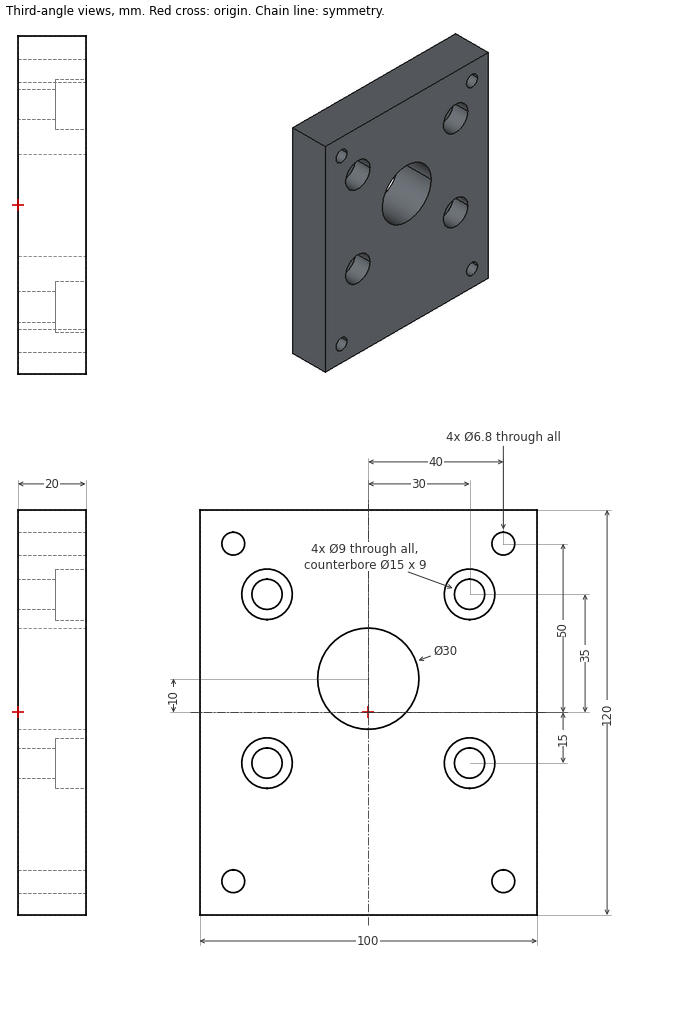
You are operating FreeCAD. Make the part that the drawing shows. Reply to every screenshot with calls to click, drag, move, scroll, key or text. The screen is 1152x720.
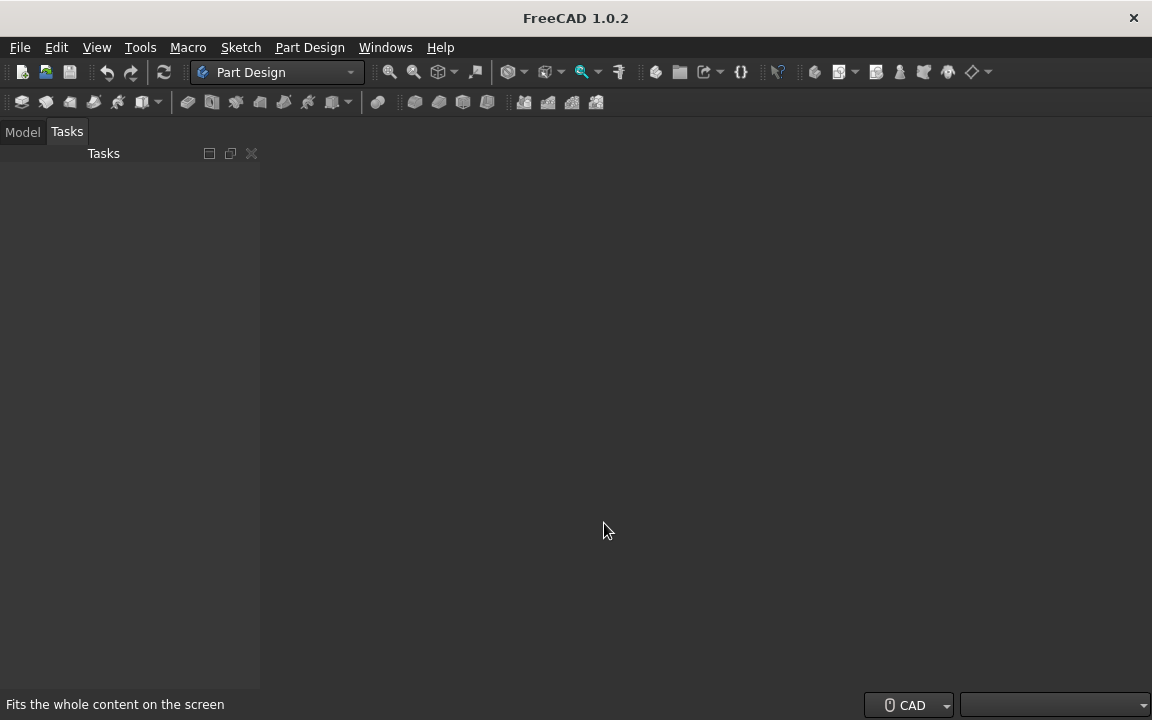
click(22, 72)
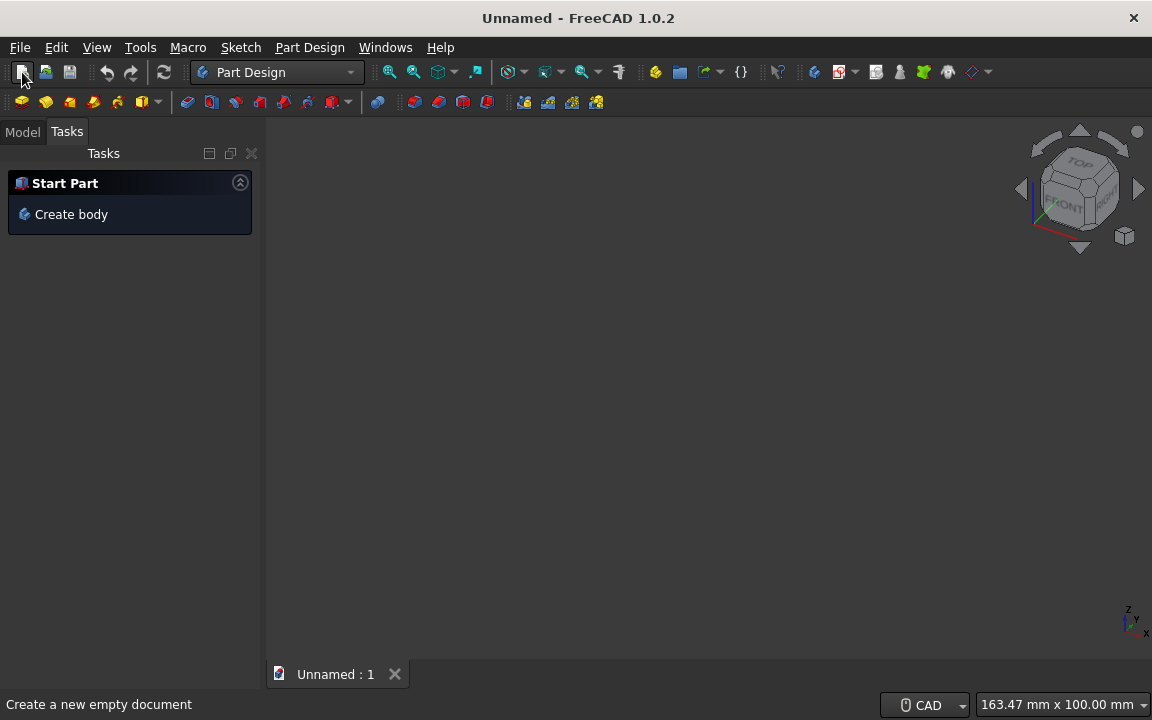
click(840, 72)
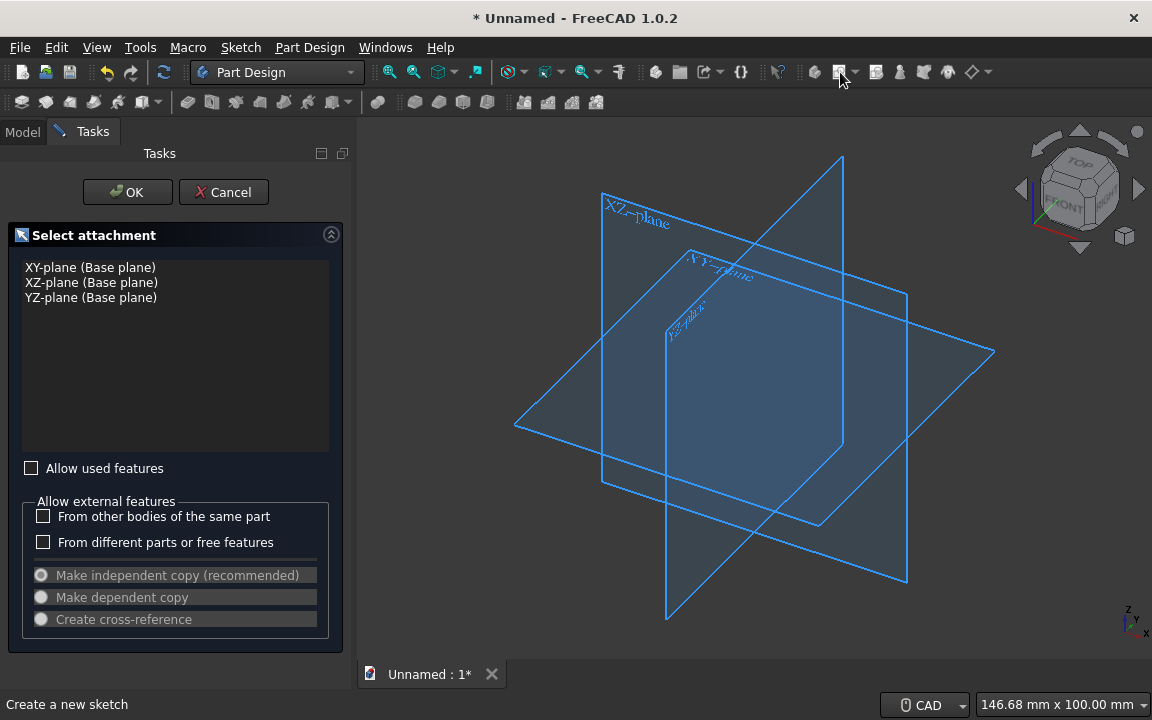
click(82, 298)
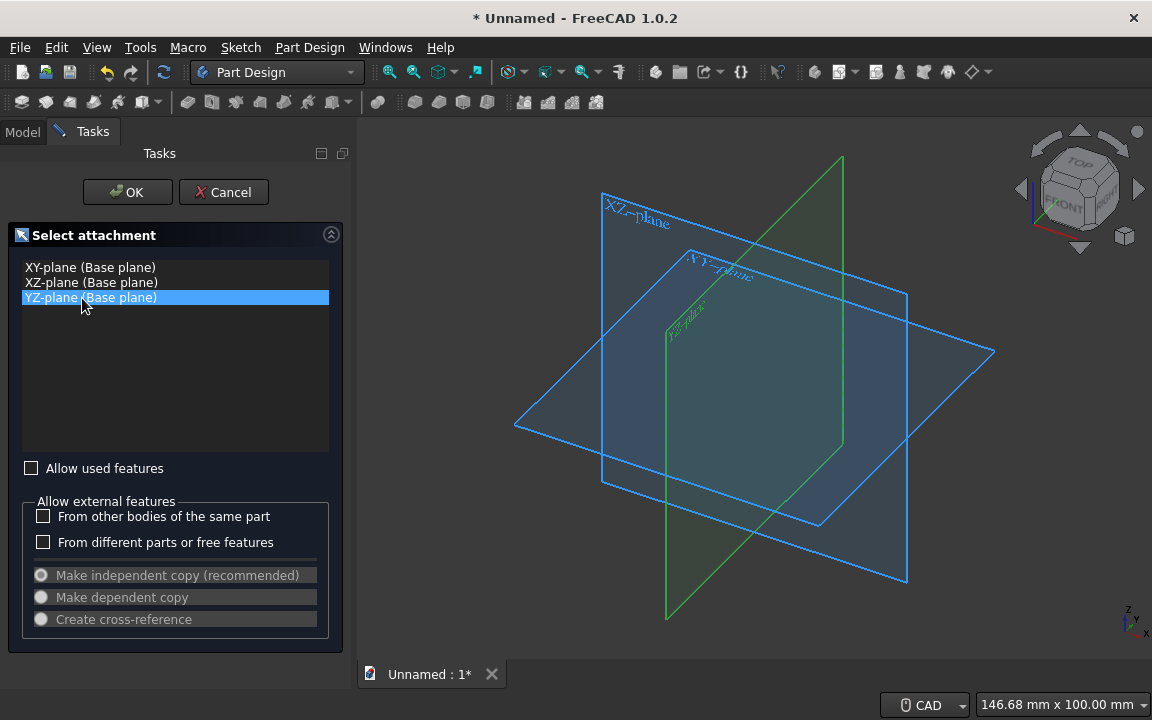
click(128, 192)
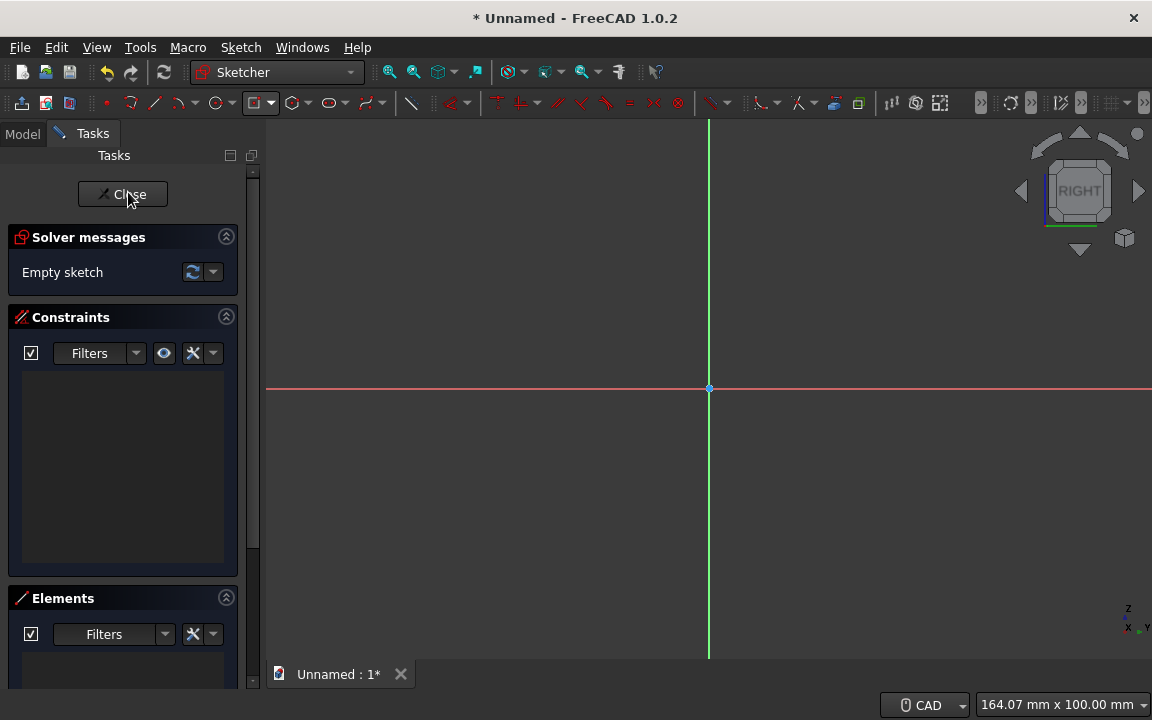
scroll(557, 389, down, 3)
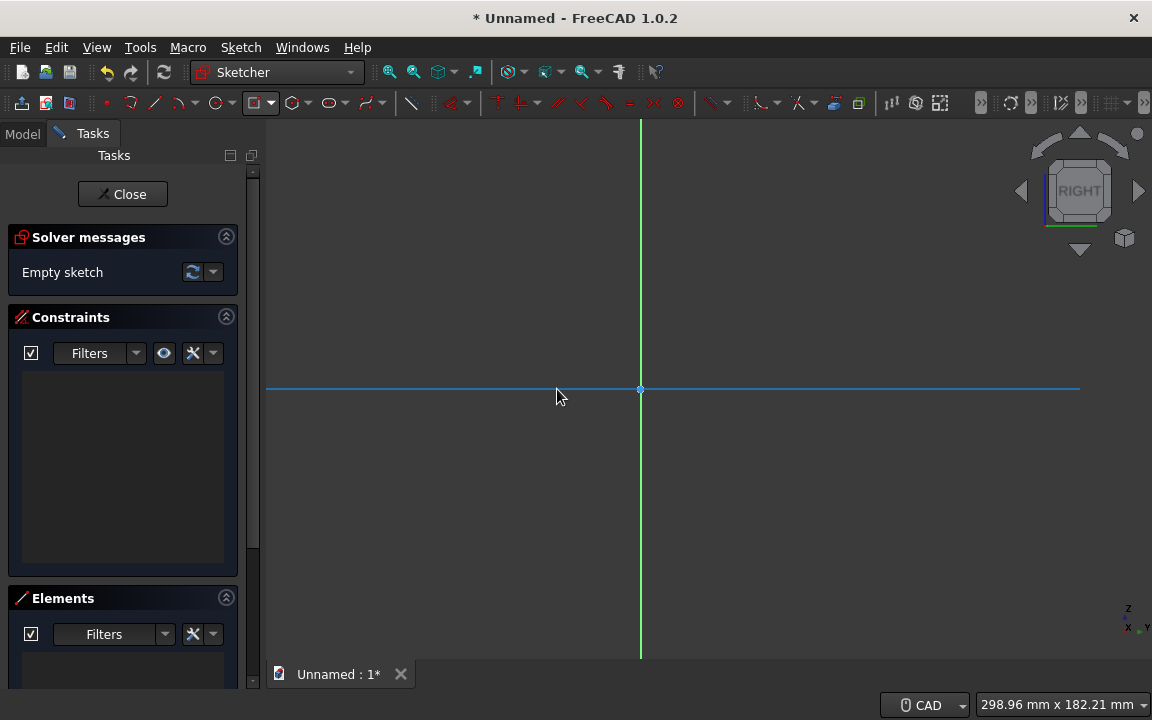
click(254, 104)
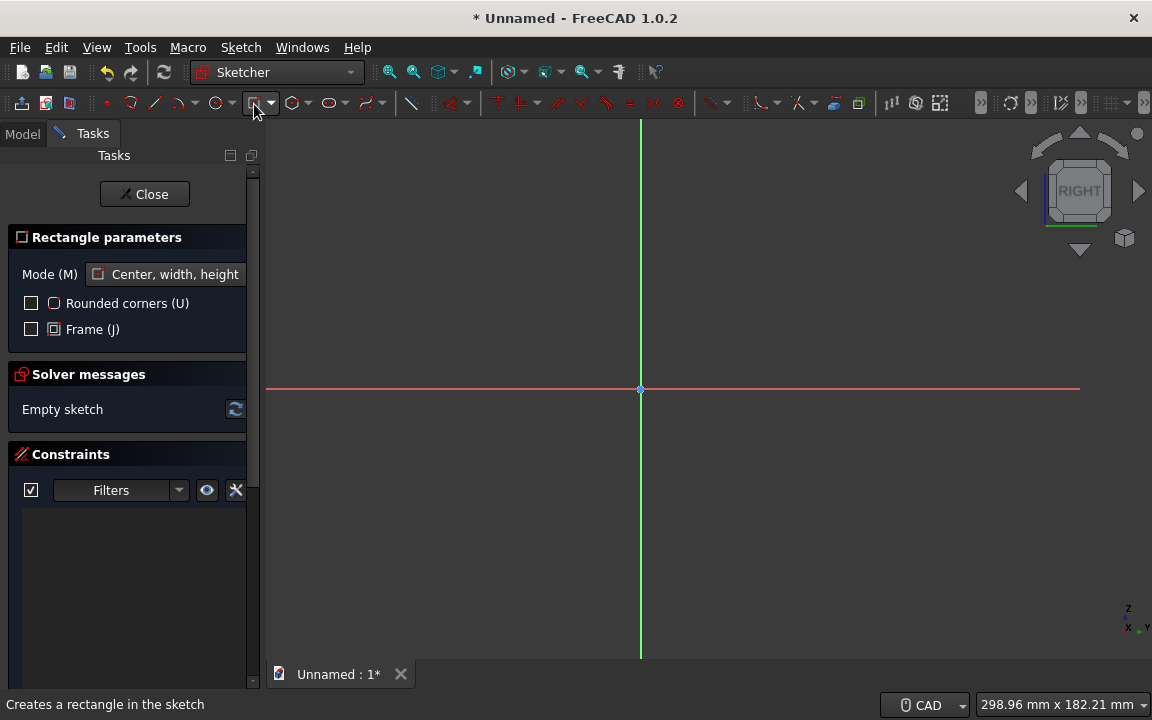
click(641, 389)
click(789, 211)
key(Escape)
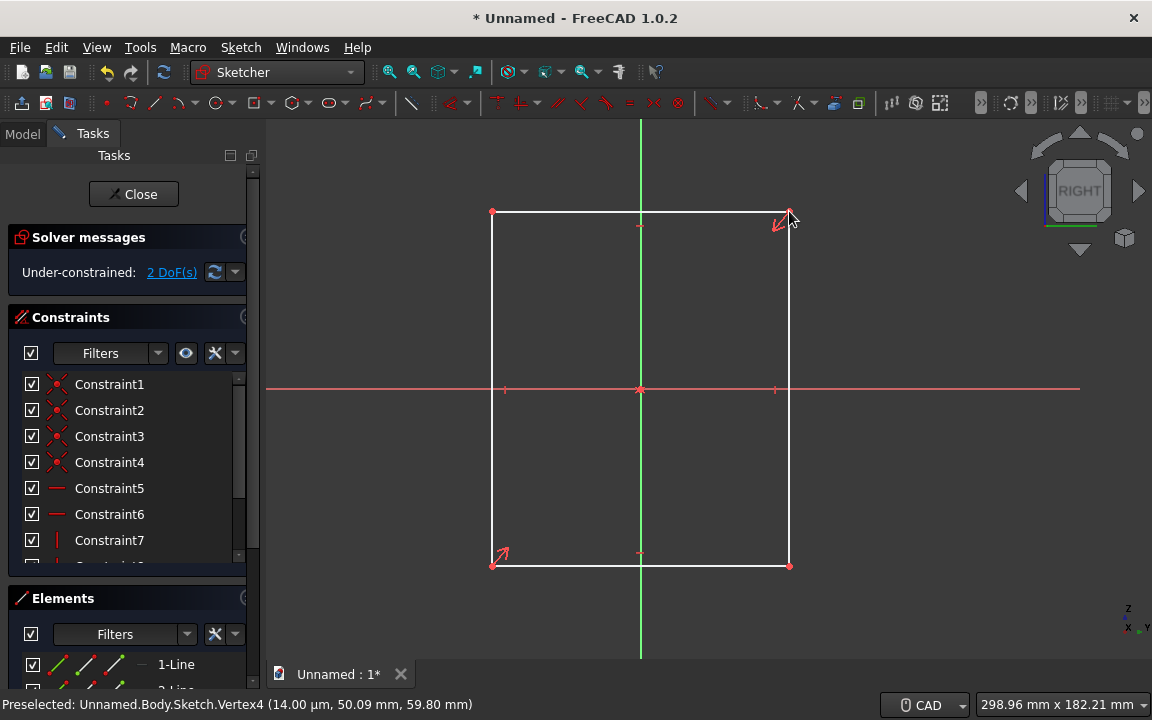
click(450, 104)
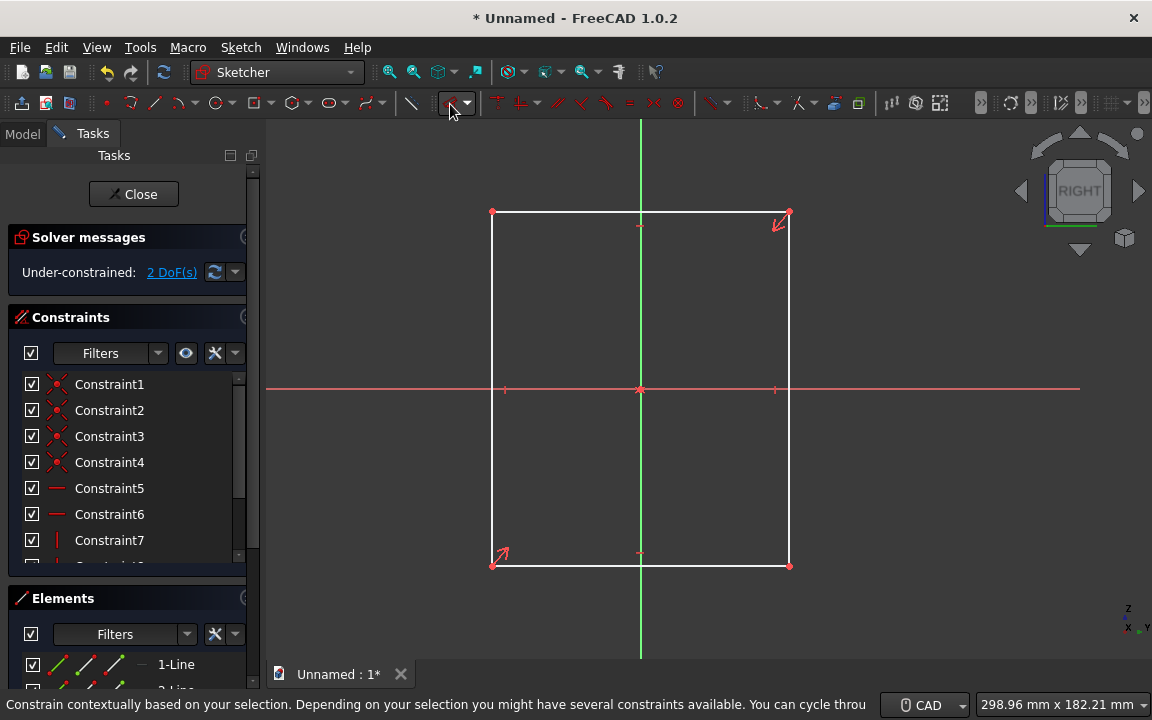
click(581, 566)
click(572, 600)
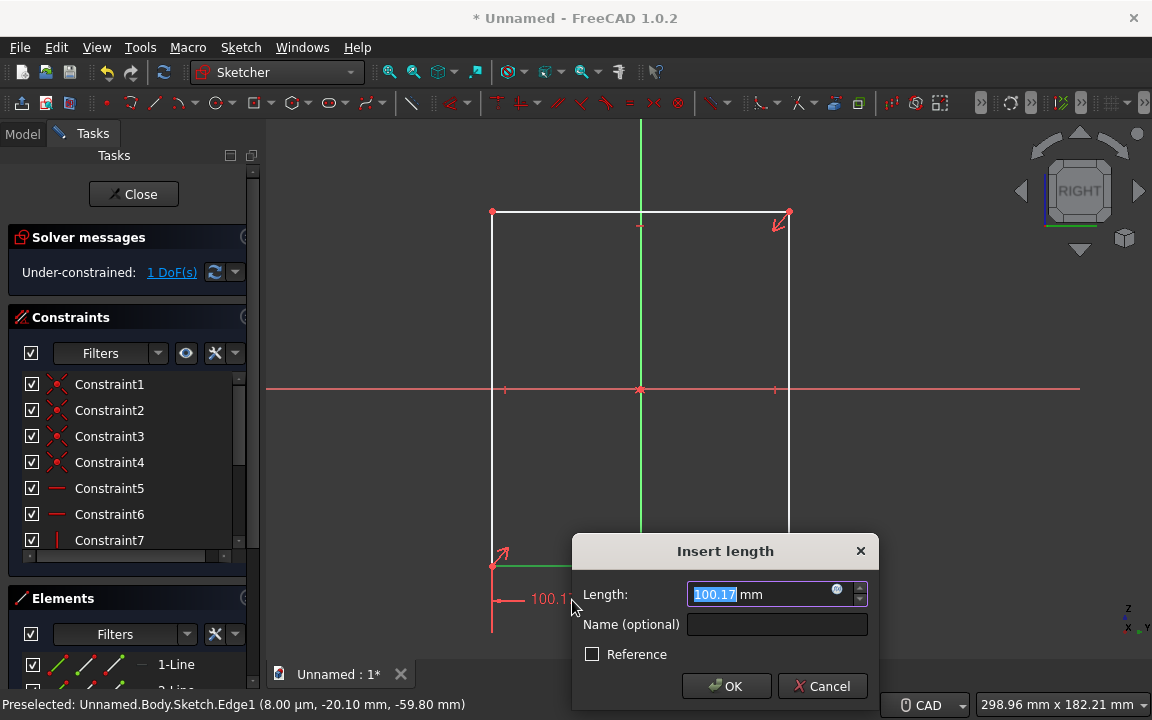
text(100)
key(Return)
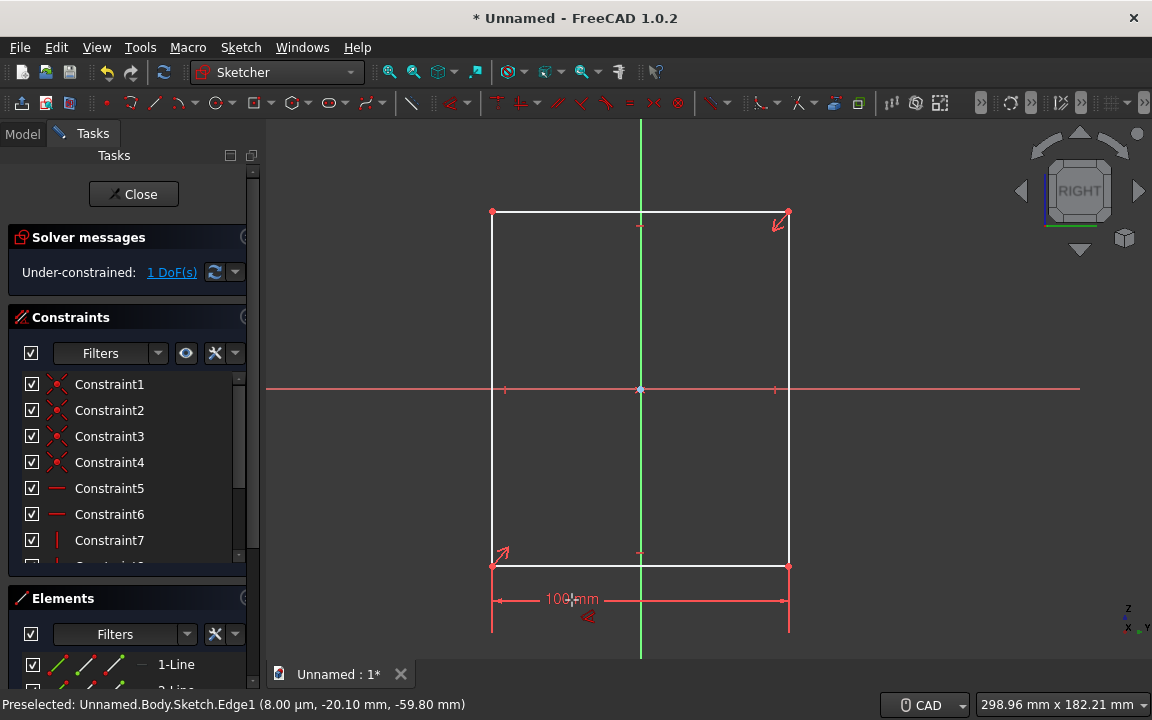
click(789, 460)
click(823, 308)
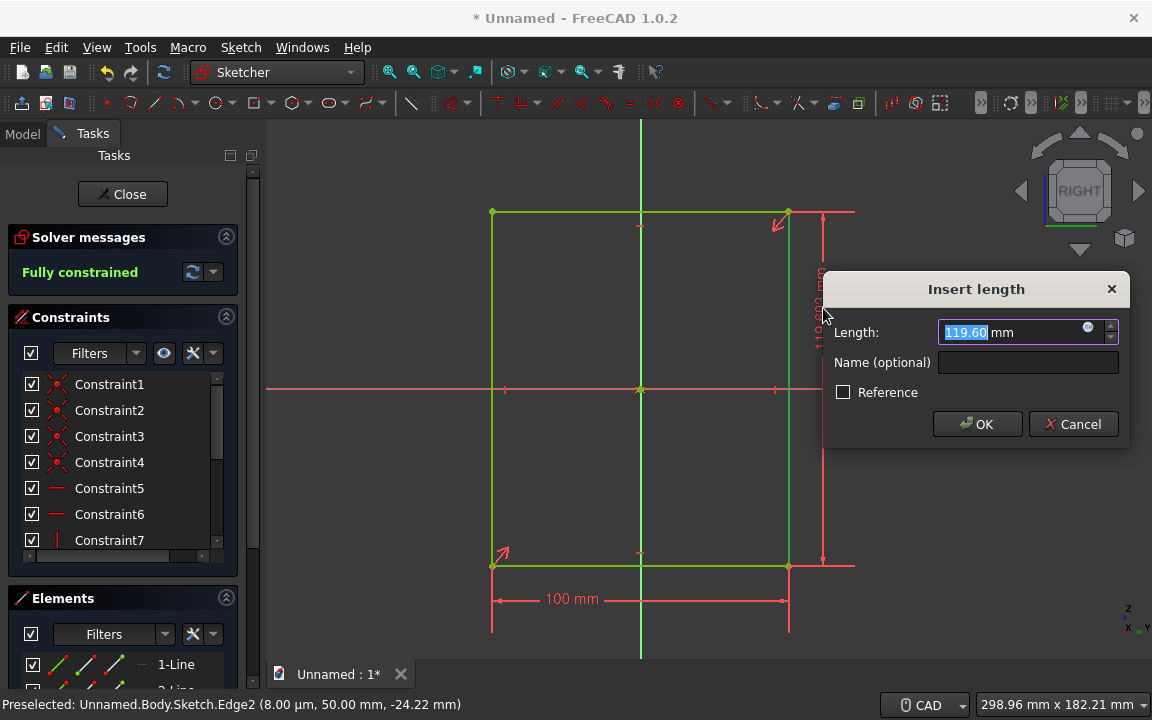
text(120)
key(Return)
key(Escape)